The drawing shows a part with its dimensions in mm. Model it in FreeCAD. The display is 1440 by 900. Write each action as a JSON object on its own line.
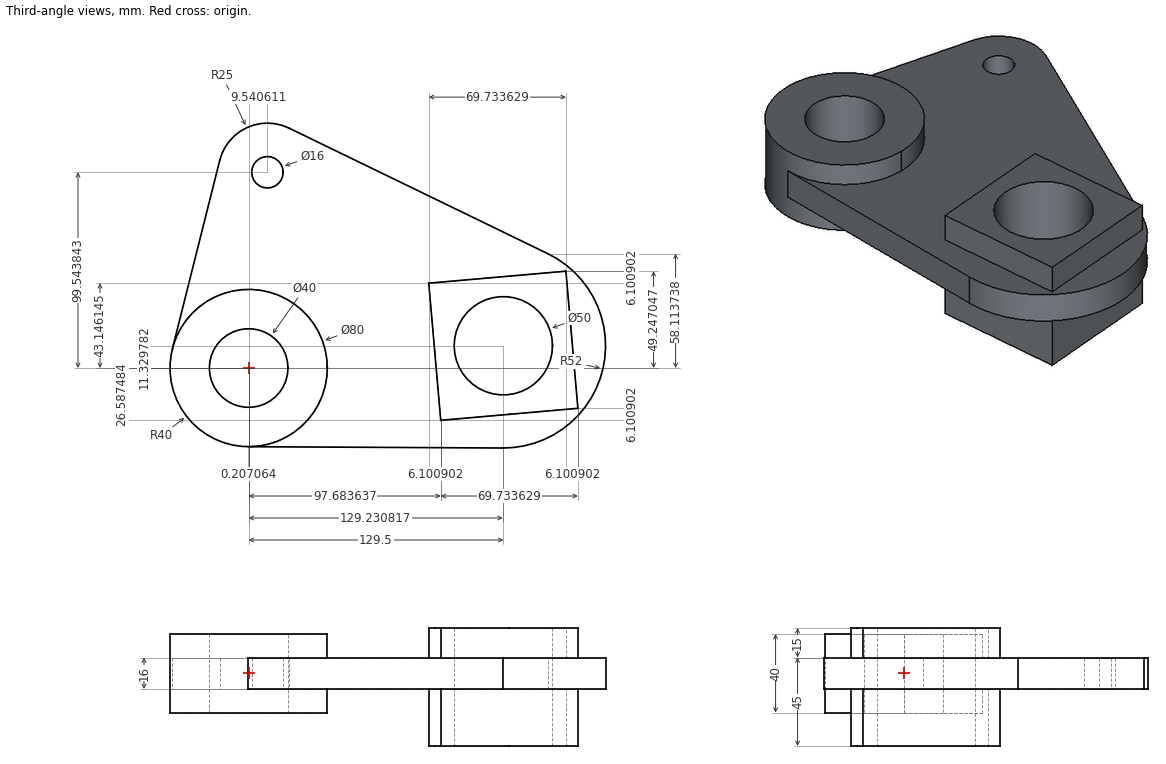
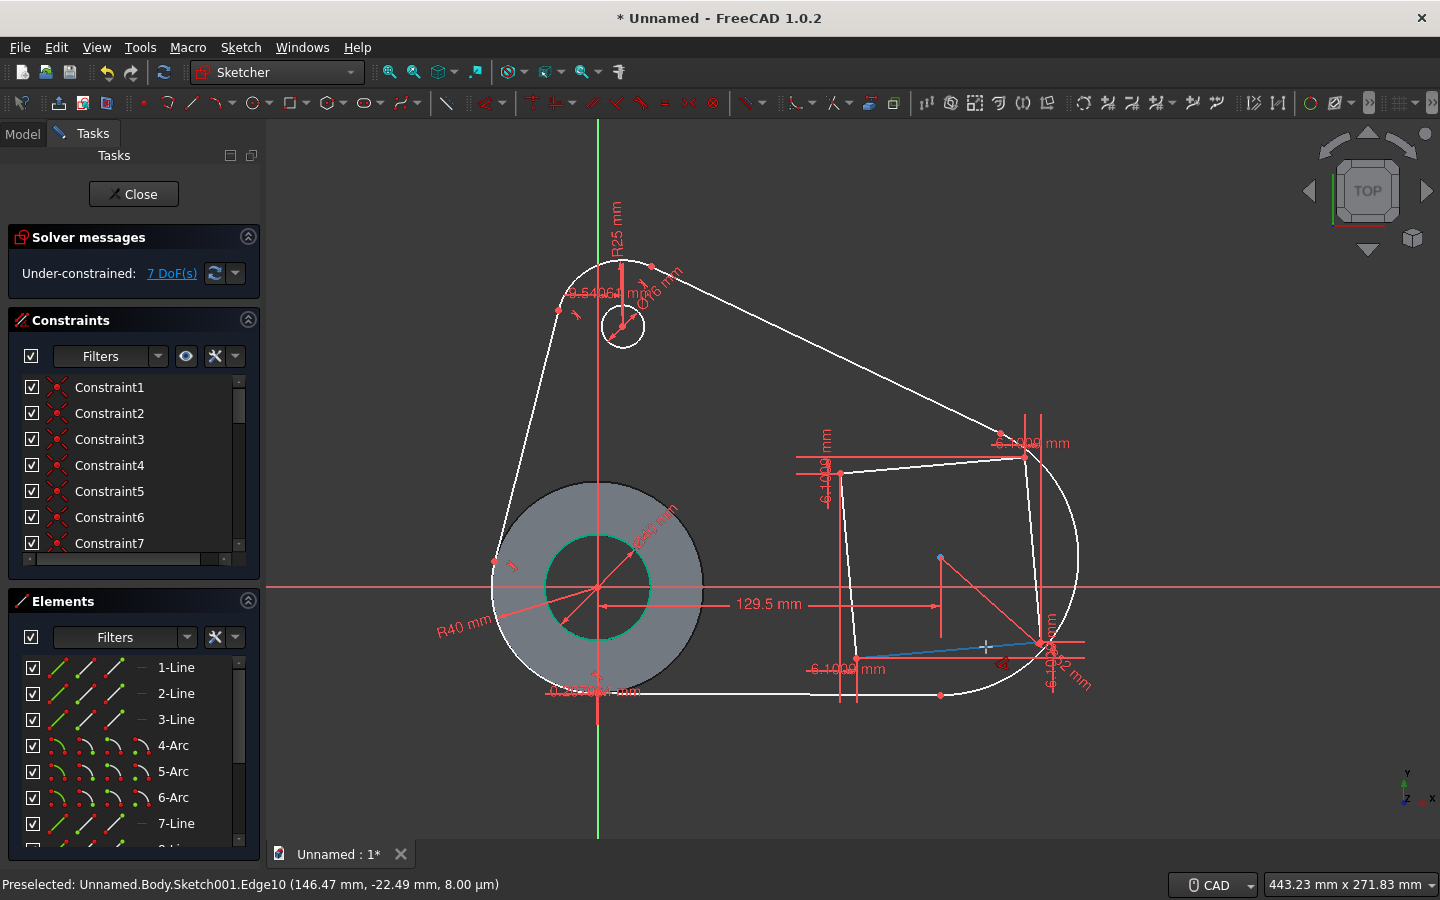
{"action": "left_click", "coordinate": [623, 327]}
{"action": "left_click", "coordinate": [564, 457]}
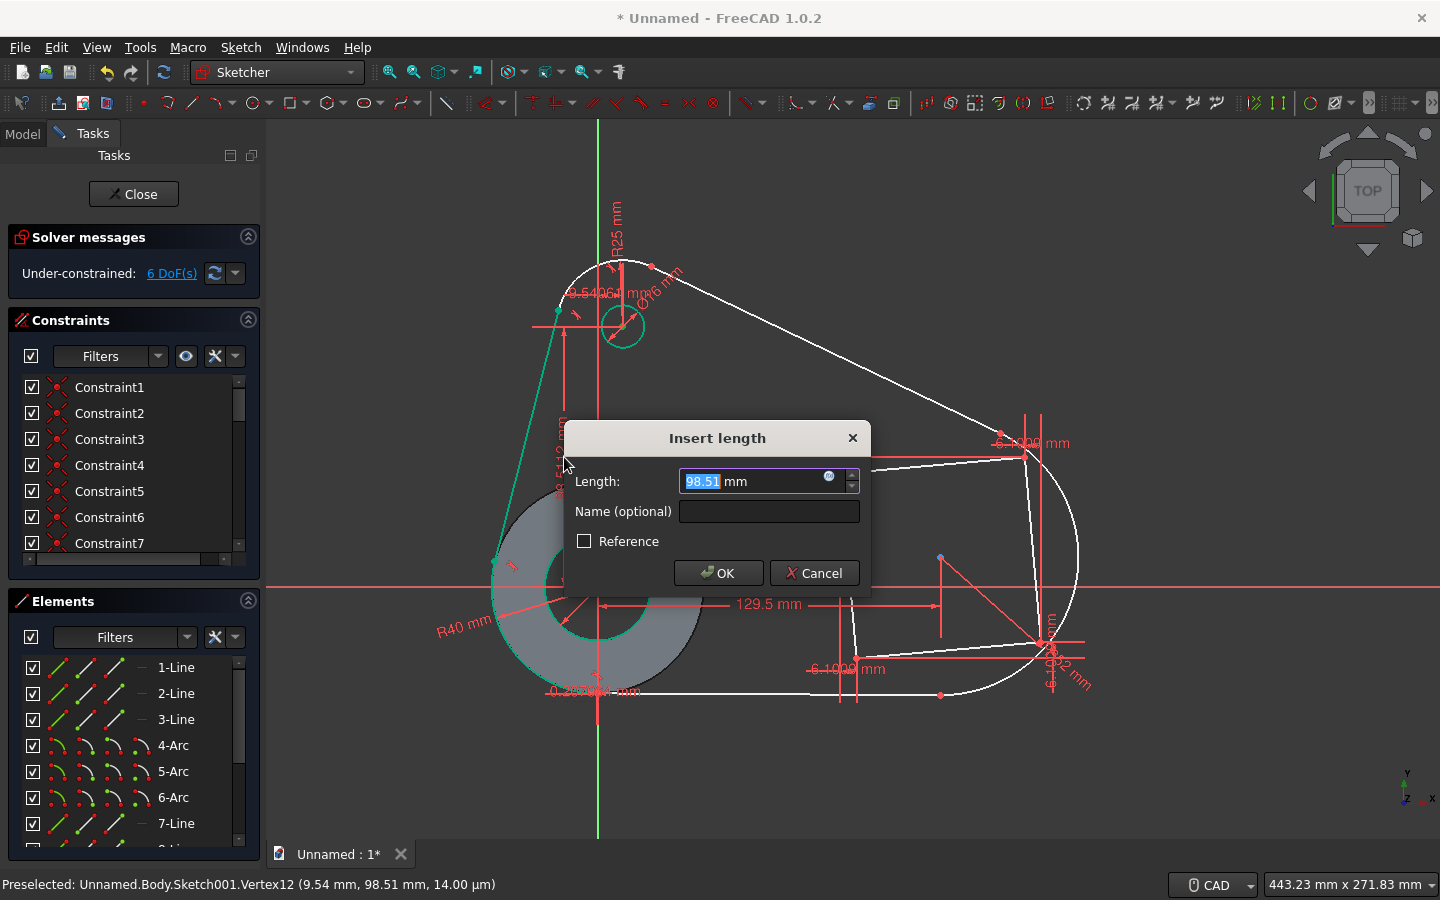
{"action": "type", "text": "99.543843"}
{"action": "key", "text": "Return"}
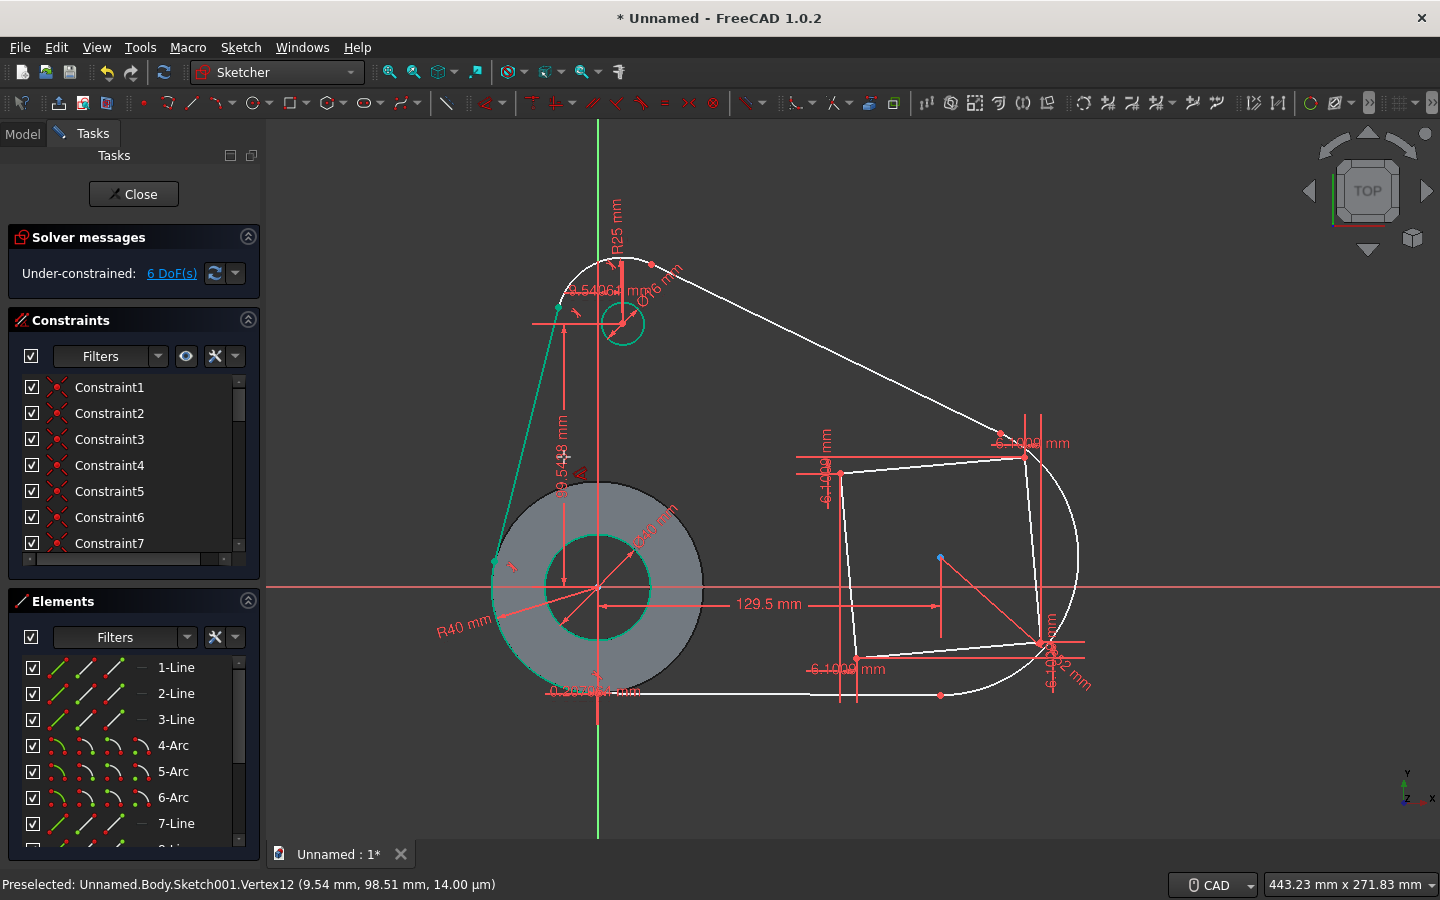
{"action": "left_click", "coordinate": [1001, 433]}
{"action": "left_click", "coordinate": [564, 510]}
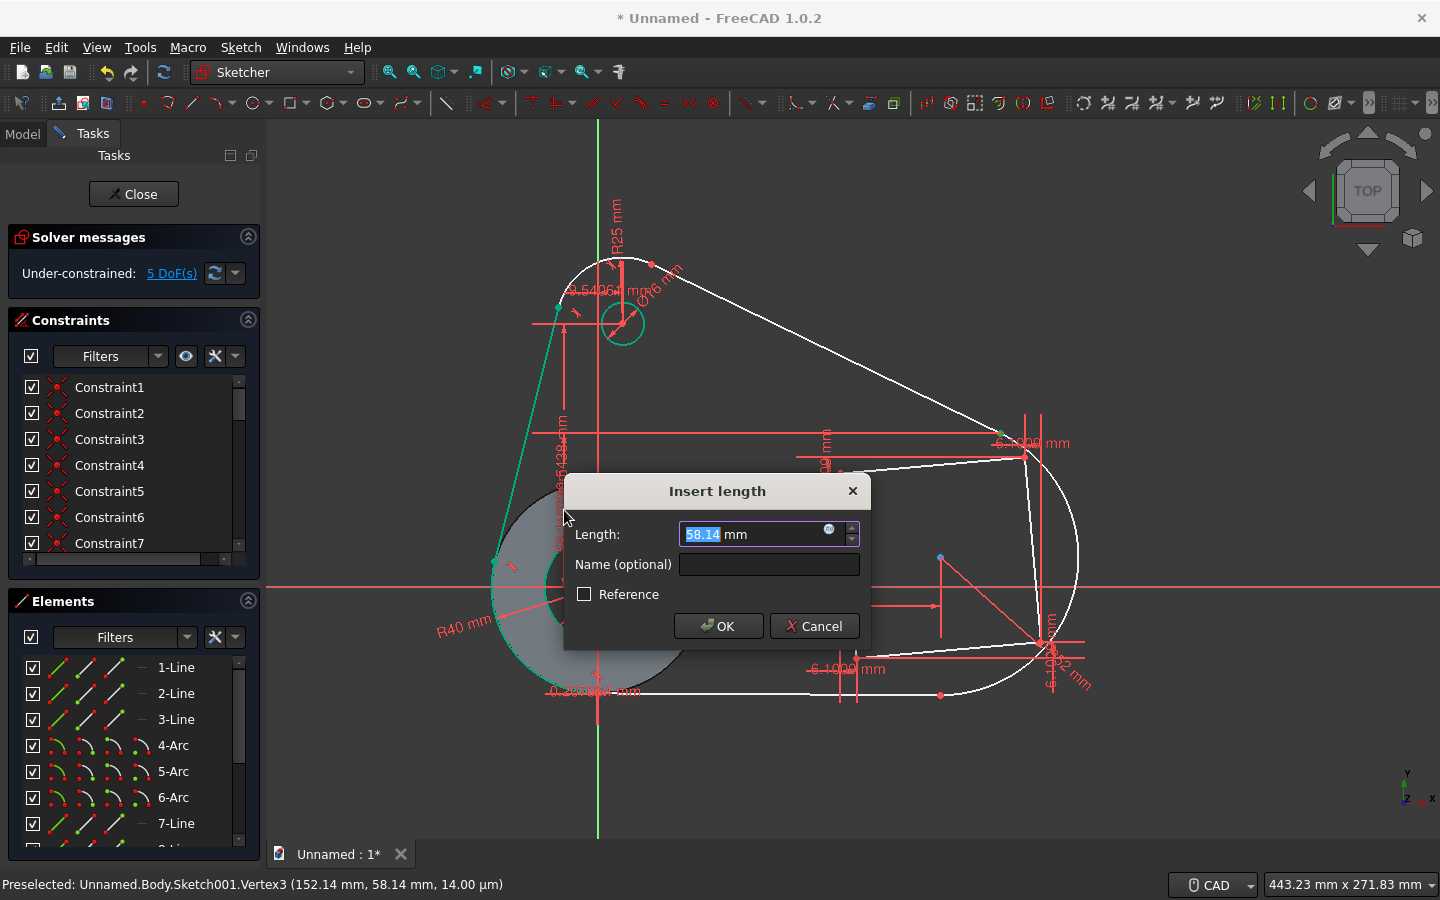
{"action": "type", "text": "58.113738"}
{"action": "key", "text": "Return"}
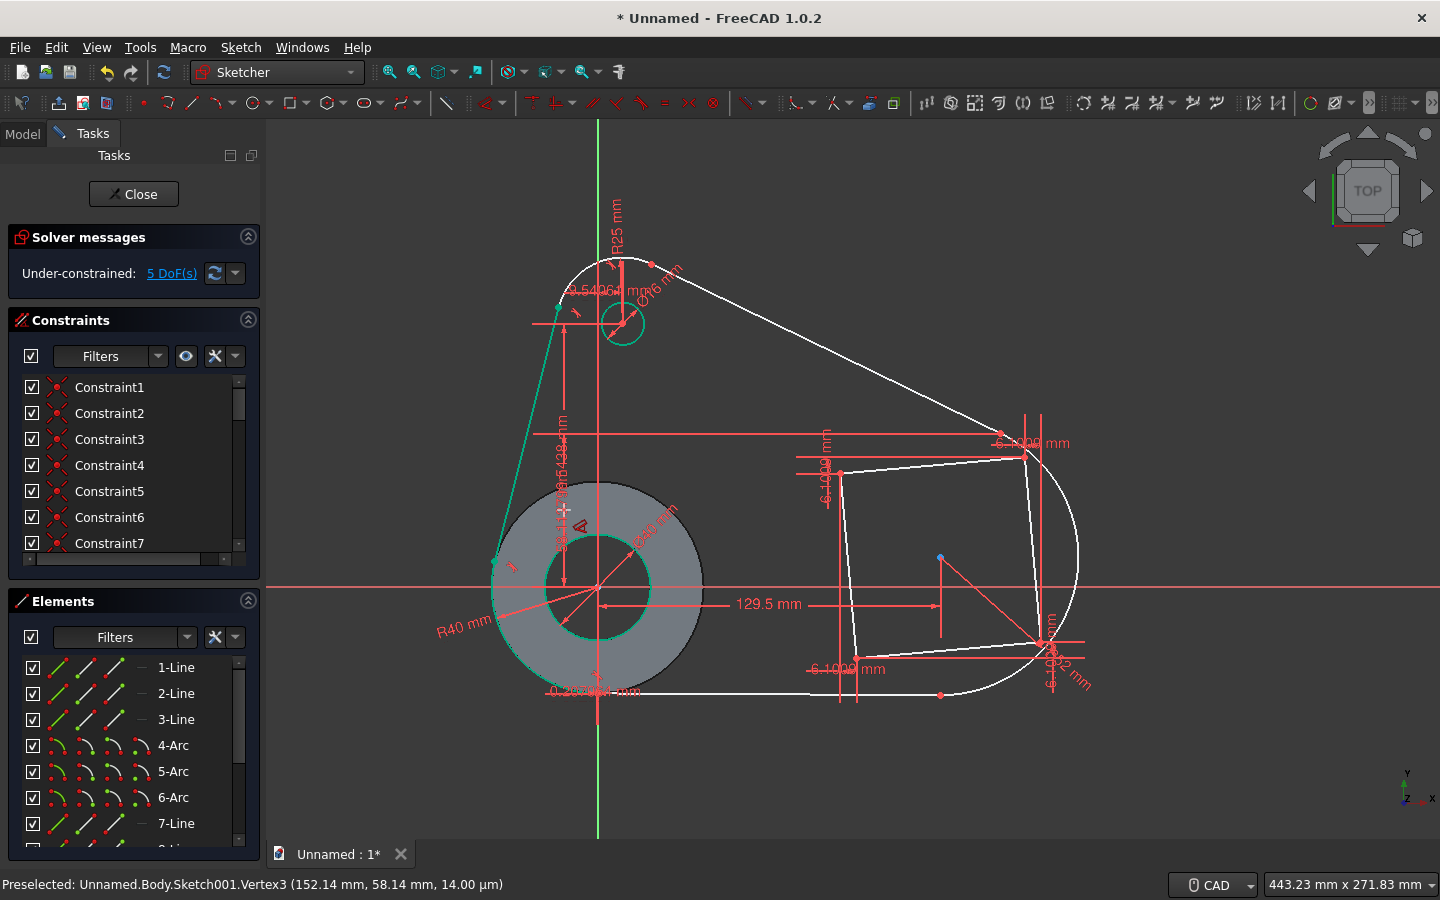
{"action": "left_click", "coordinate": [857, 658]}
{"action": "left_click", "coordinate": [727, 553]}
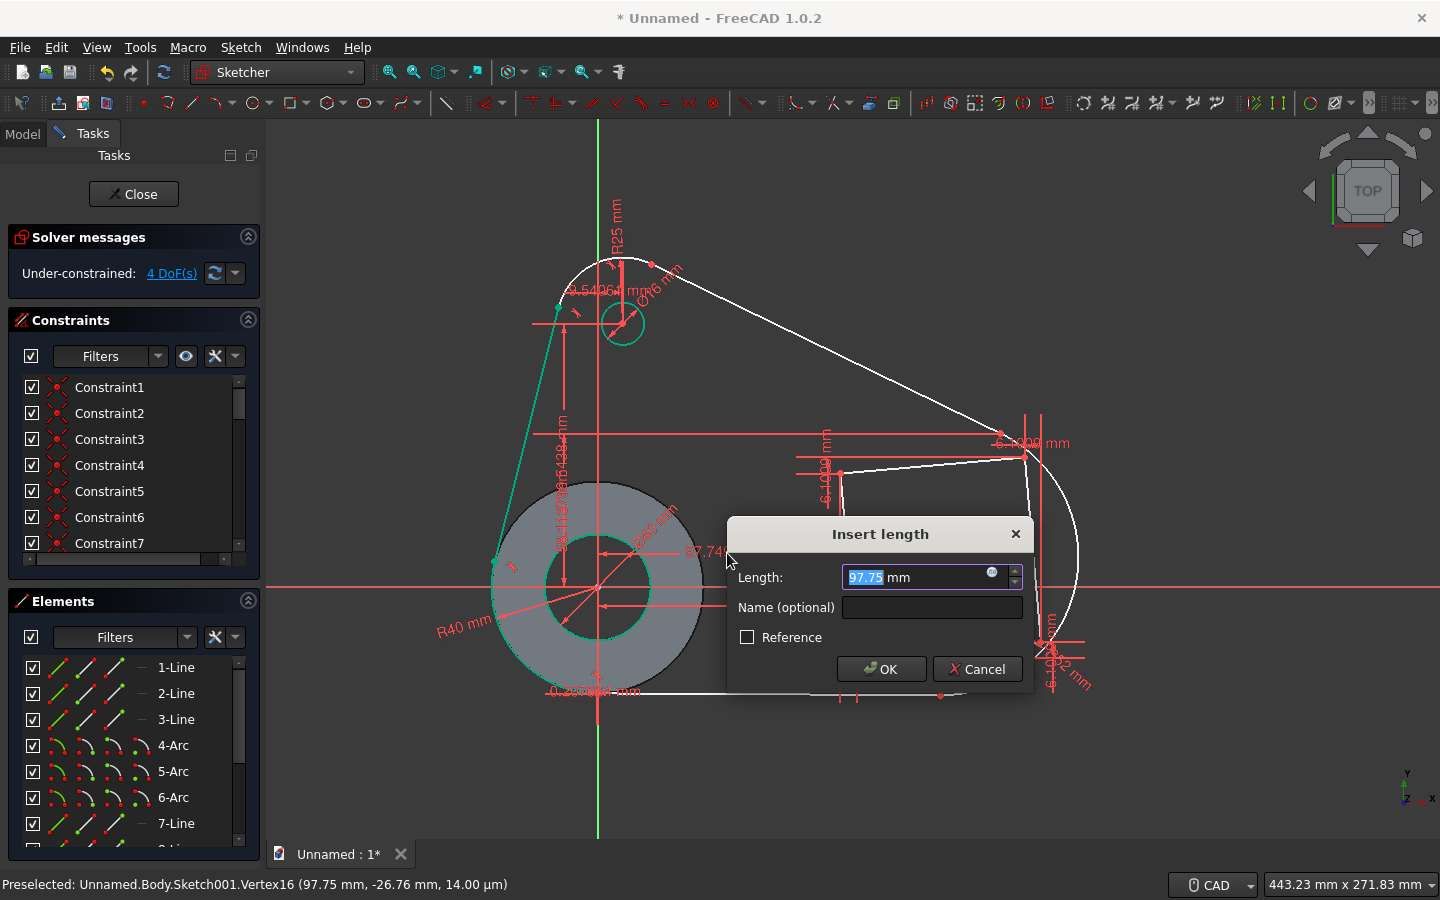
{"action": "type", "text": "97.683637"}
{"action": "key", "text": "Return"}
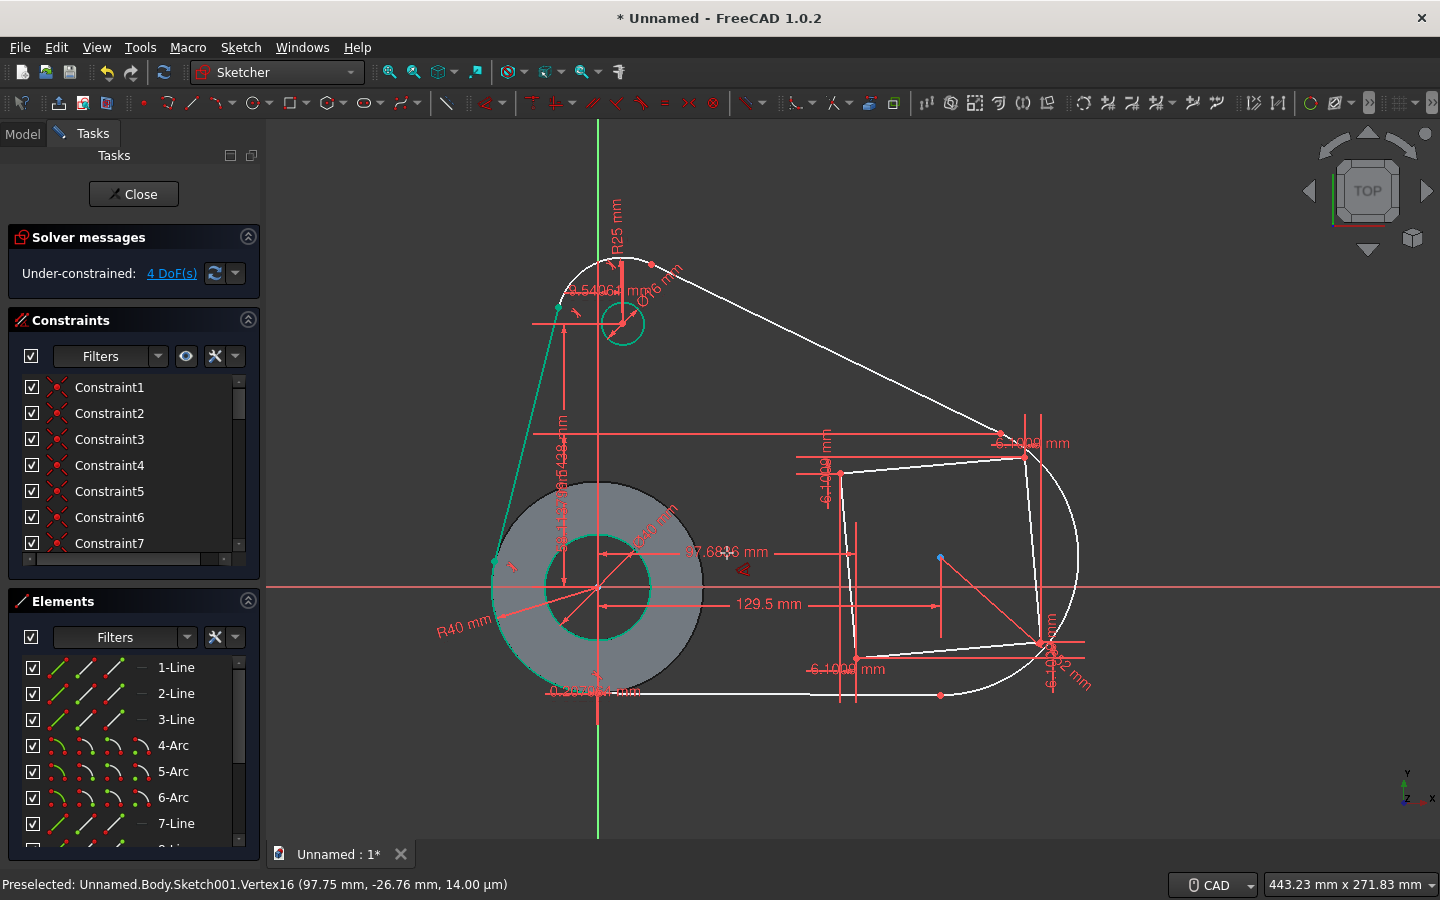
{"action": "left_click", "coordinate": [856, 658]}
{"action": "left_click", "coordinate": [564, 607]}